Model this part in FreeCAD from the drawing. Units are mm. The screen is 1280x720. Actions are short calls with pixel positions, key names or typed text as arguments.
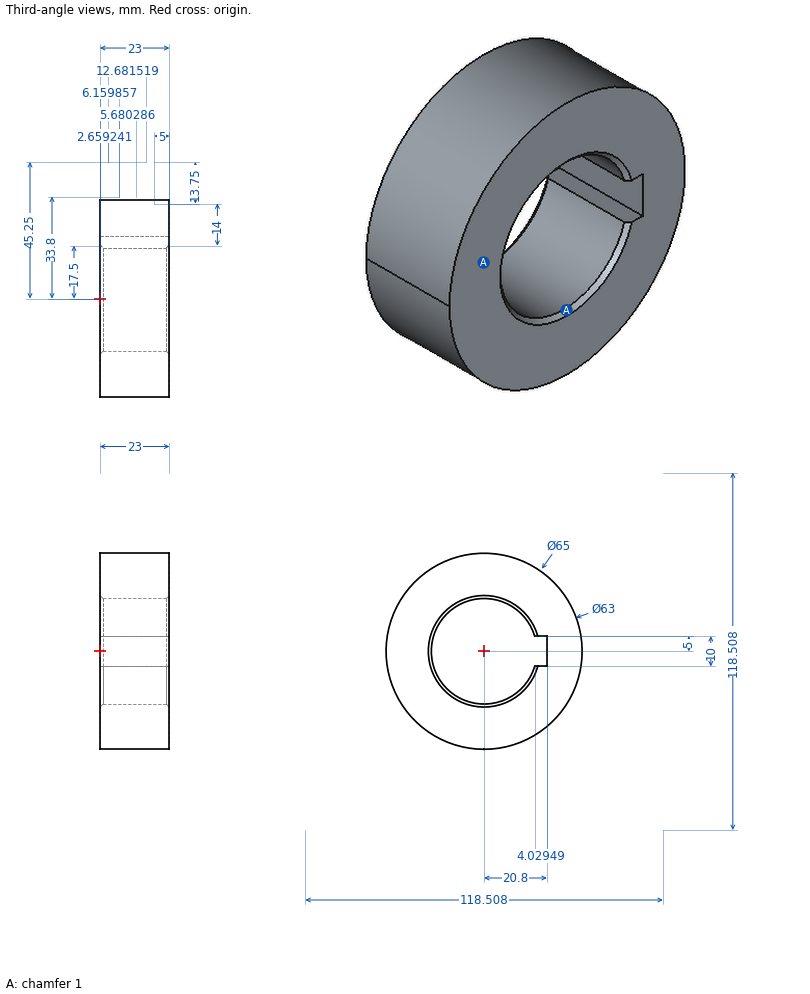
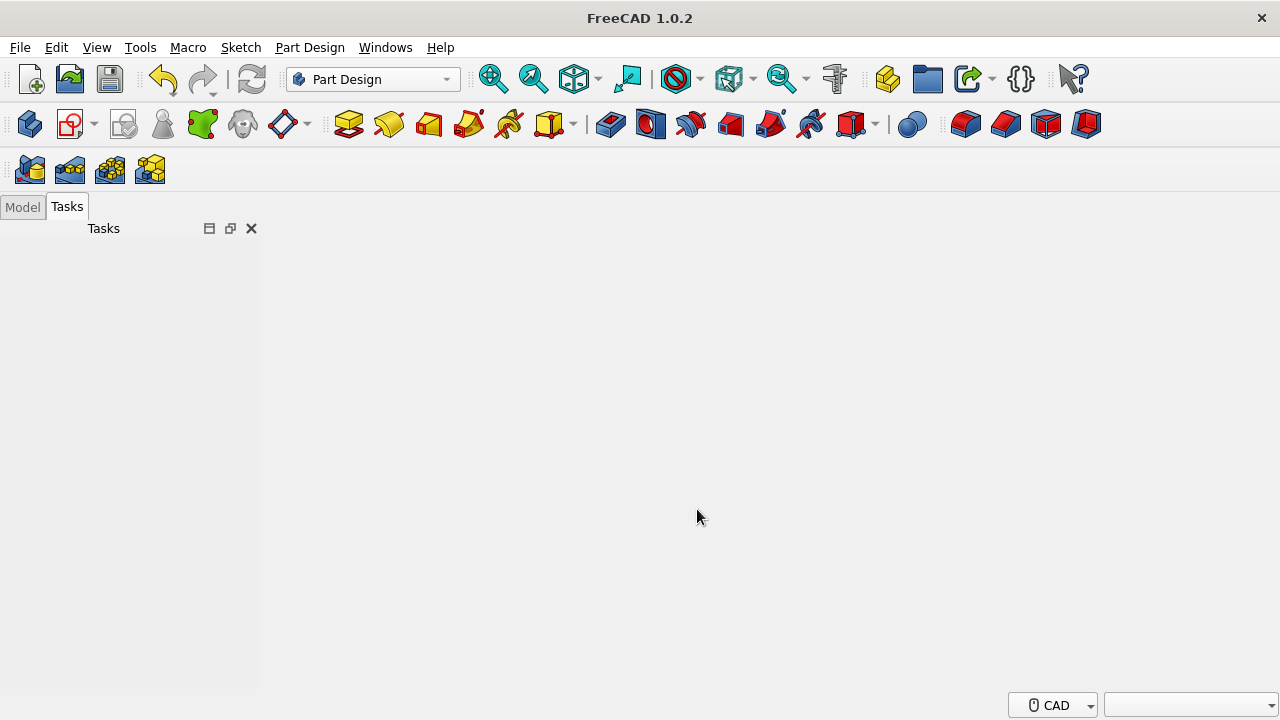
click(30, 80)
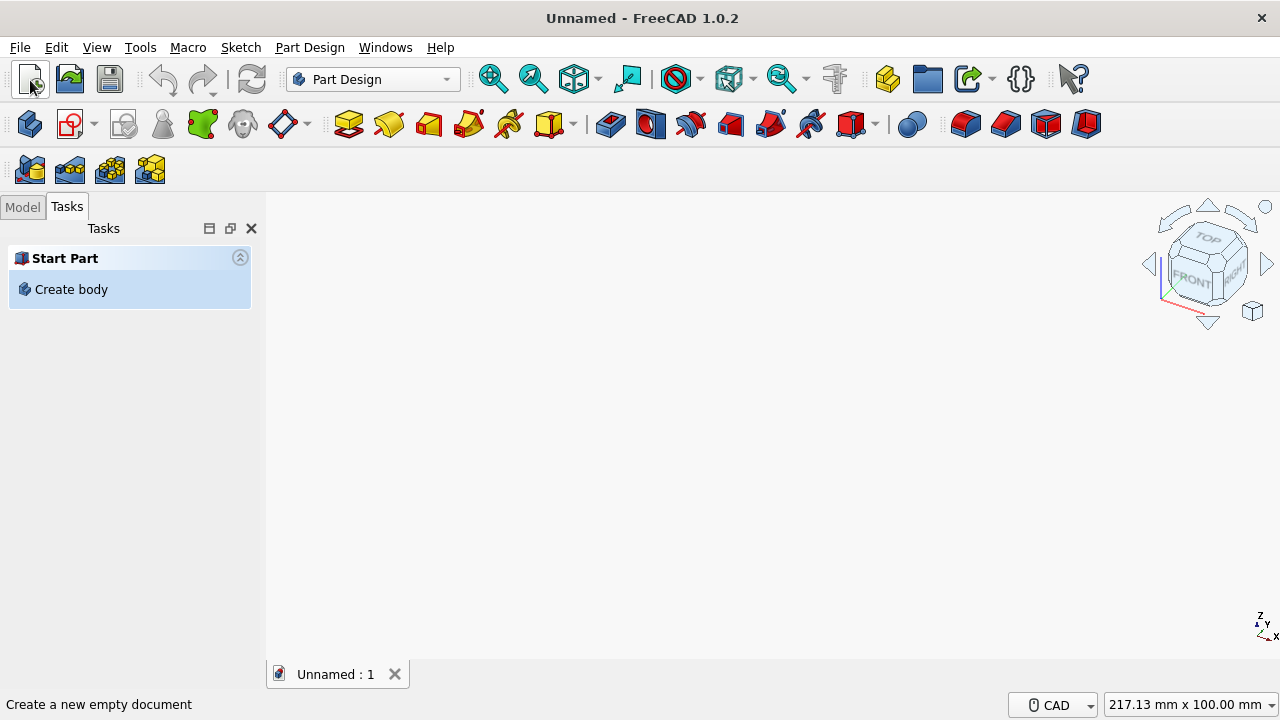
click(70, 124)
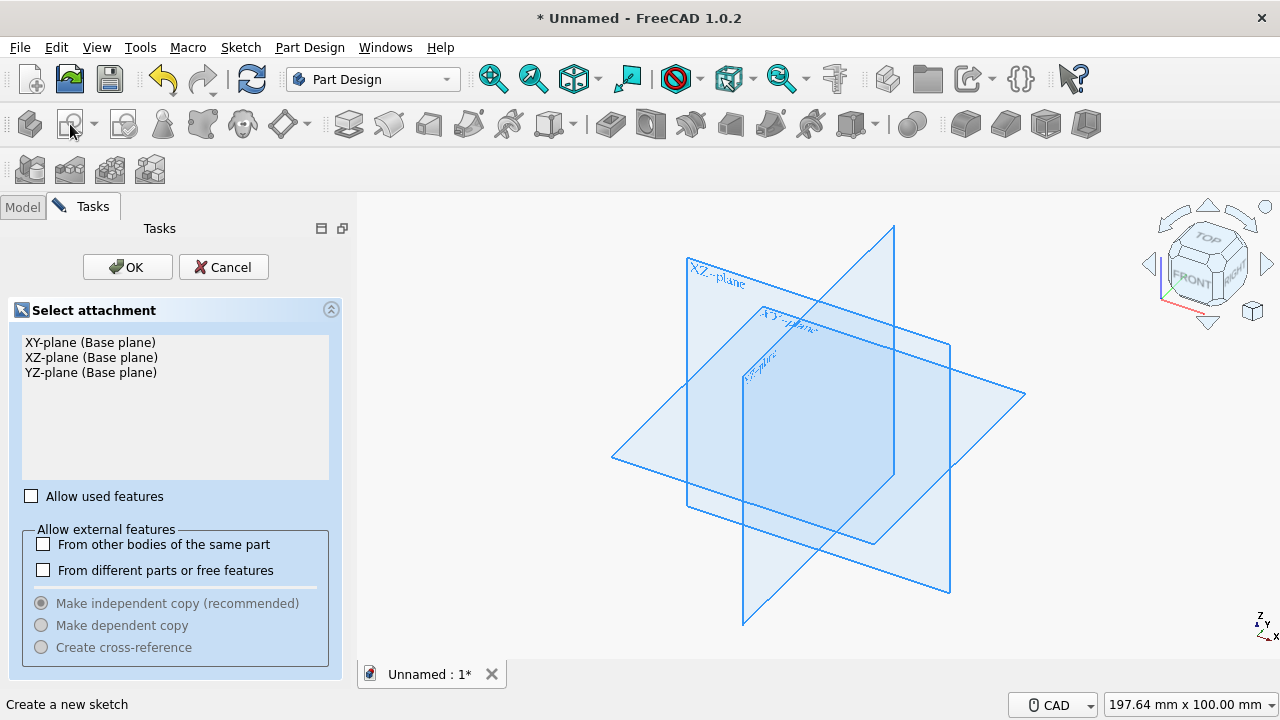
click(82, 342)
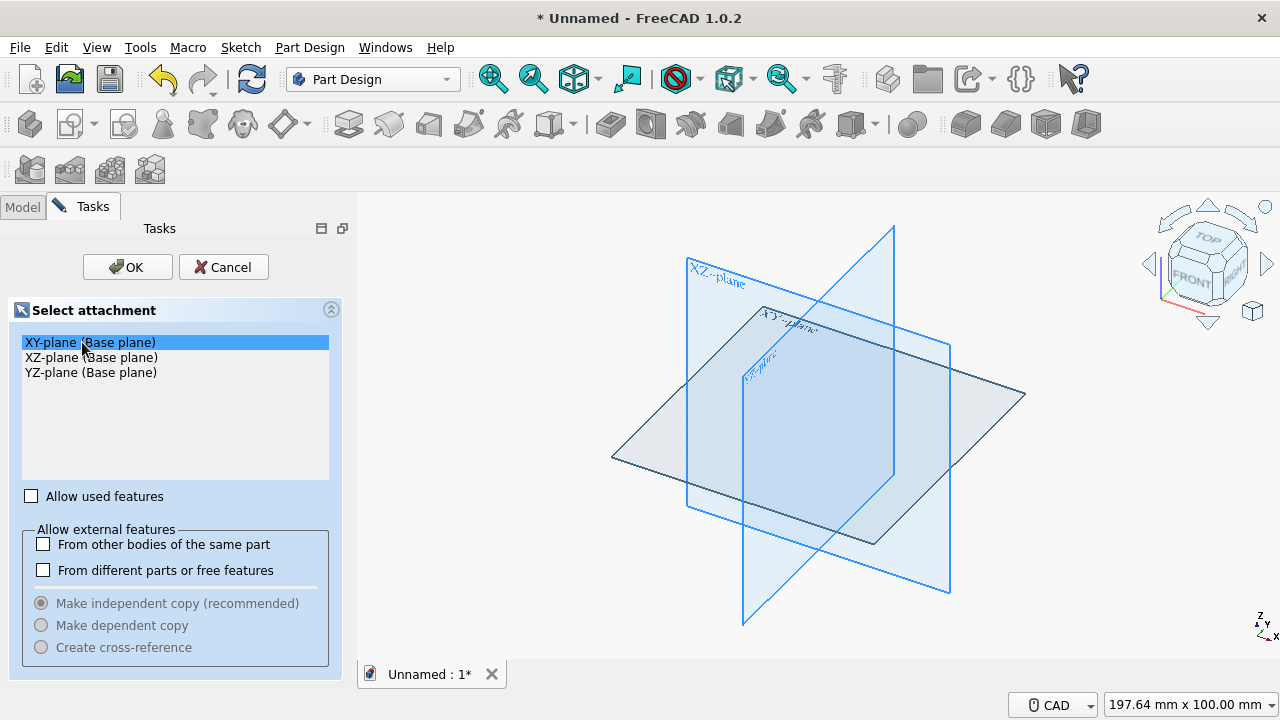
click(128, 267)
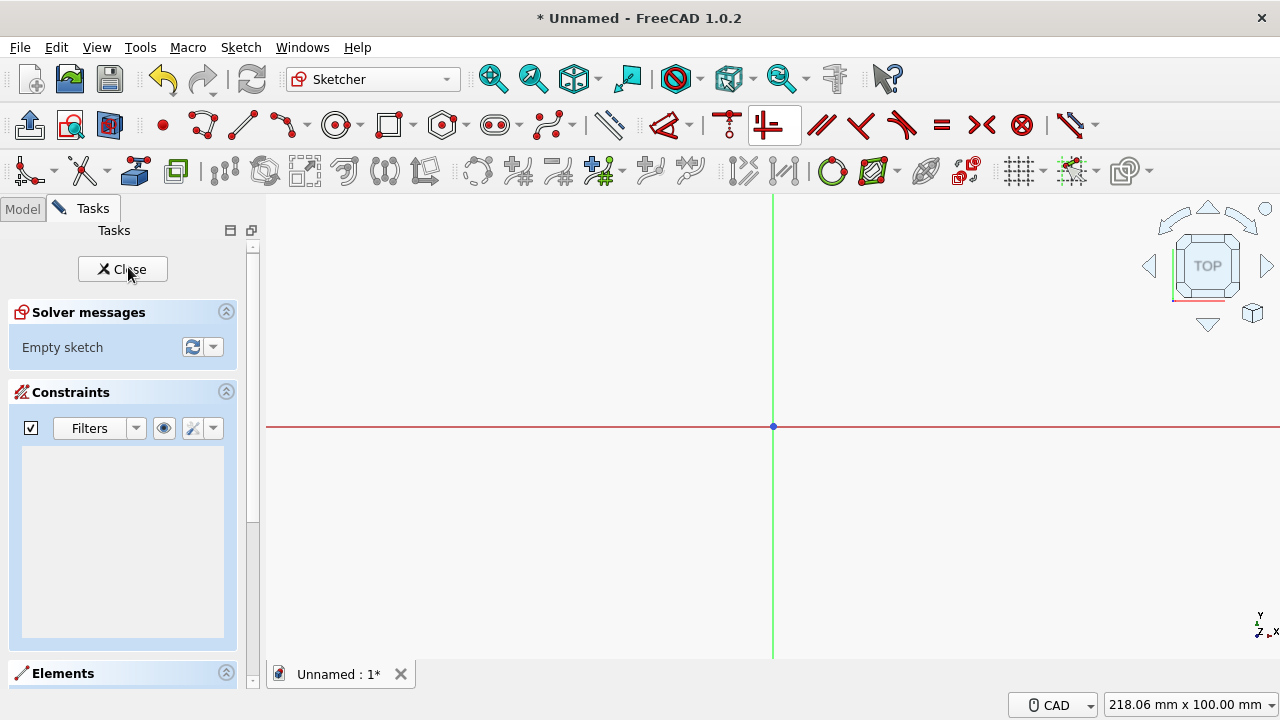
scroll(294, 631, down, 1)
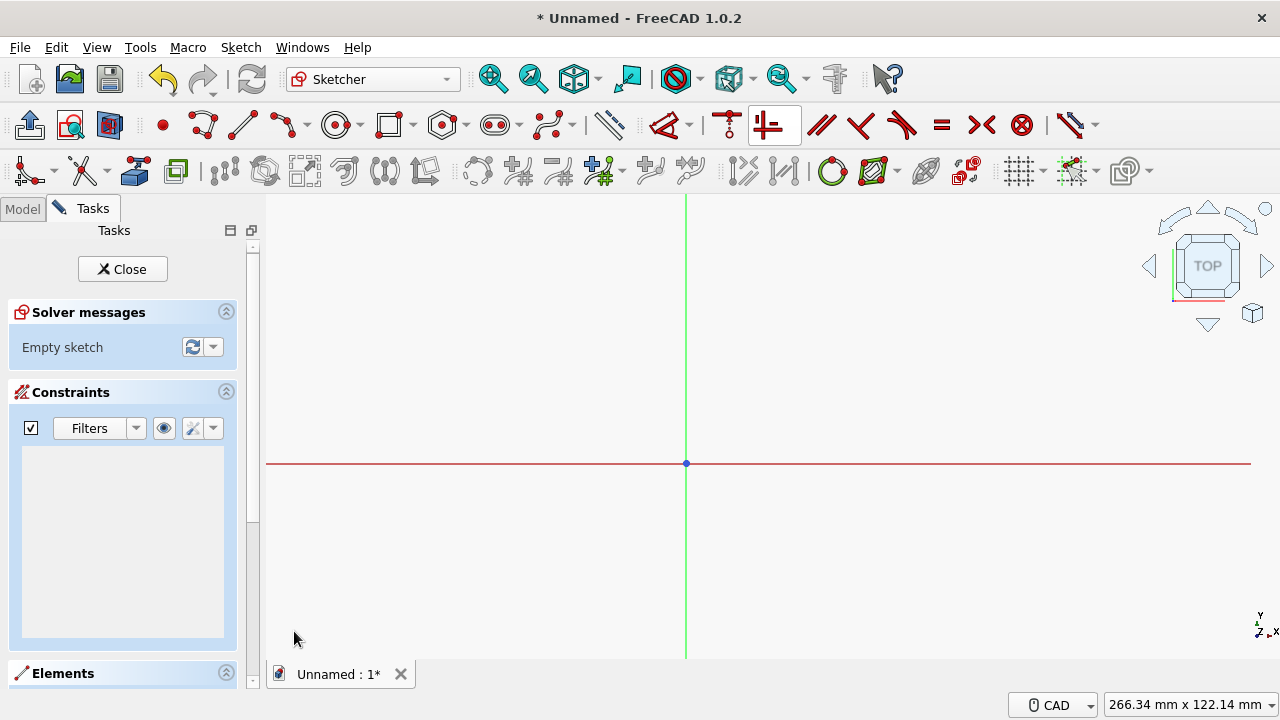
scroll(761, 318, up, 3)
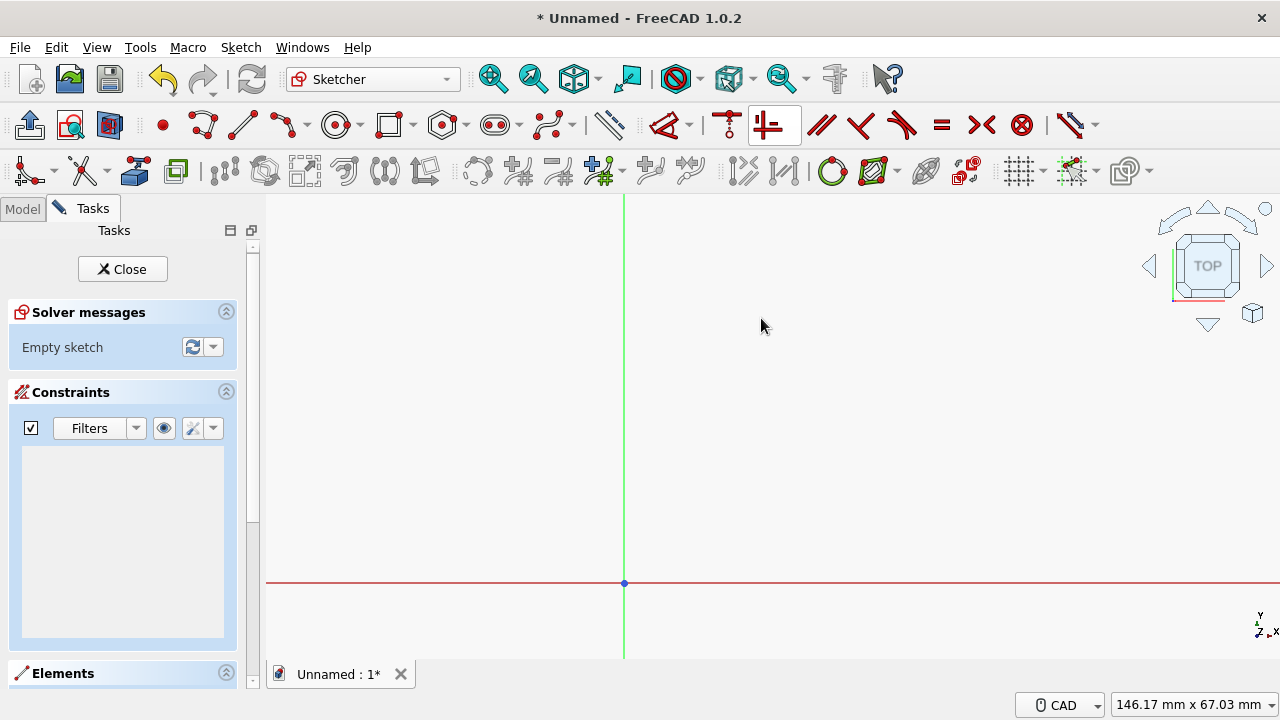
key(g)
key(m)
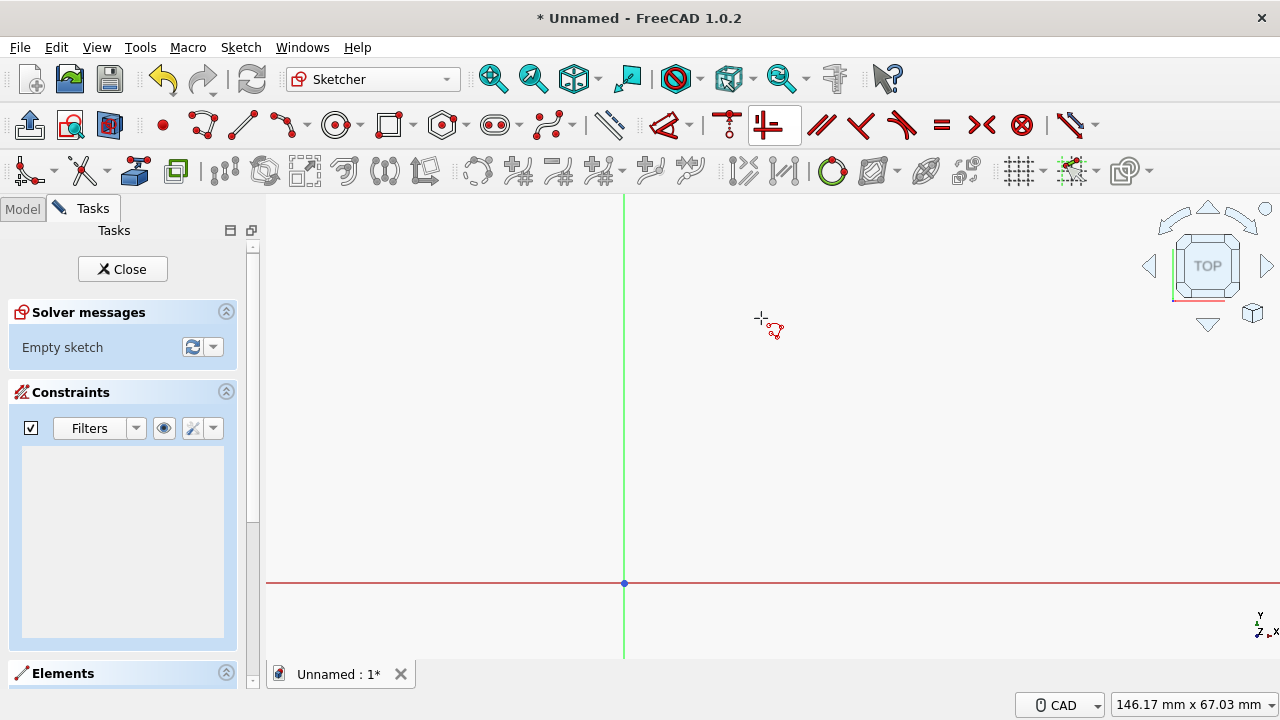
click(624, 462)
click(784, 462)
click(784, 365)
click(749, 365)
click(749, 269)
click(633, 269)
click(624, 463)
key(Escape)
key(Escape)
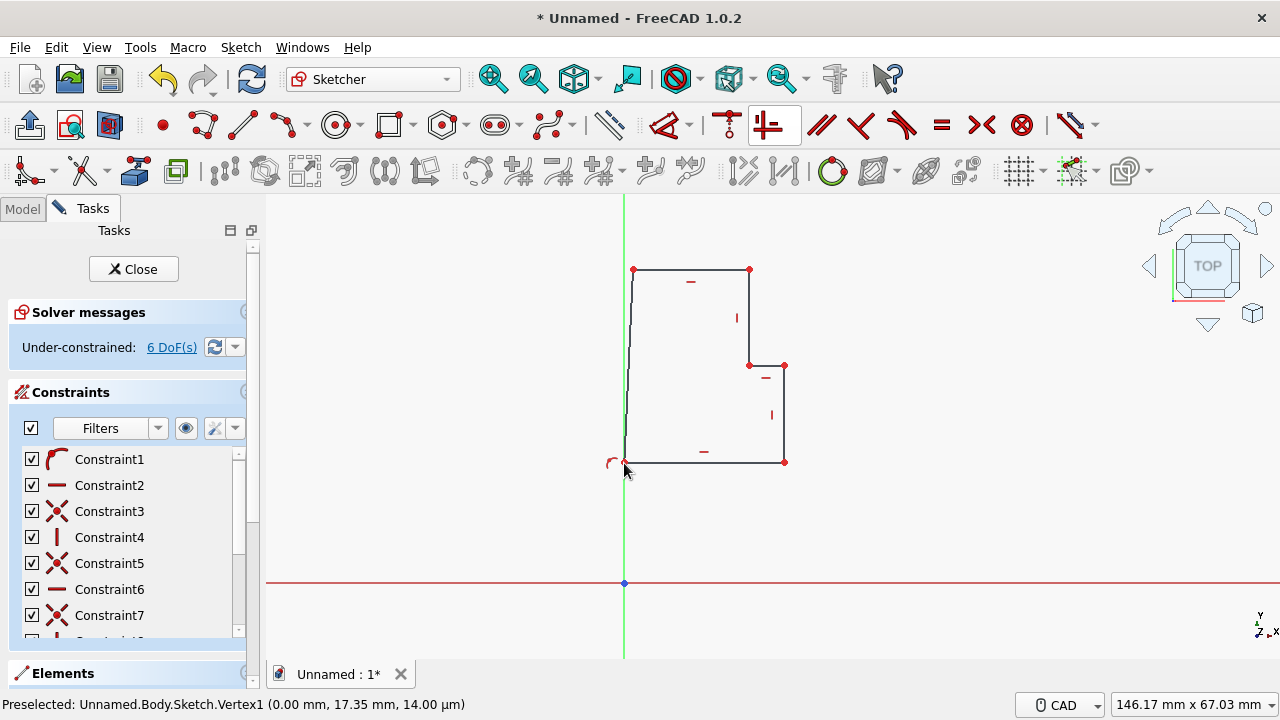
click(627, 405)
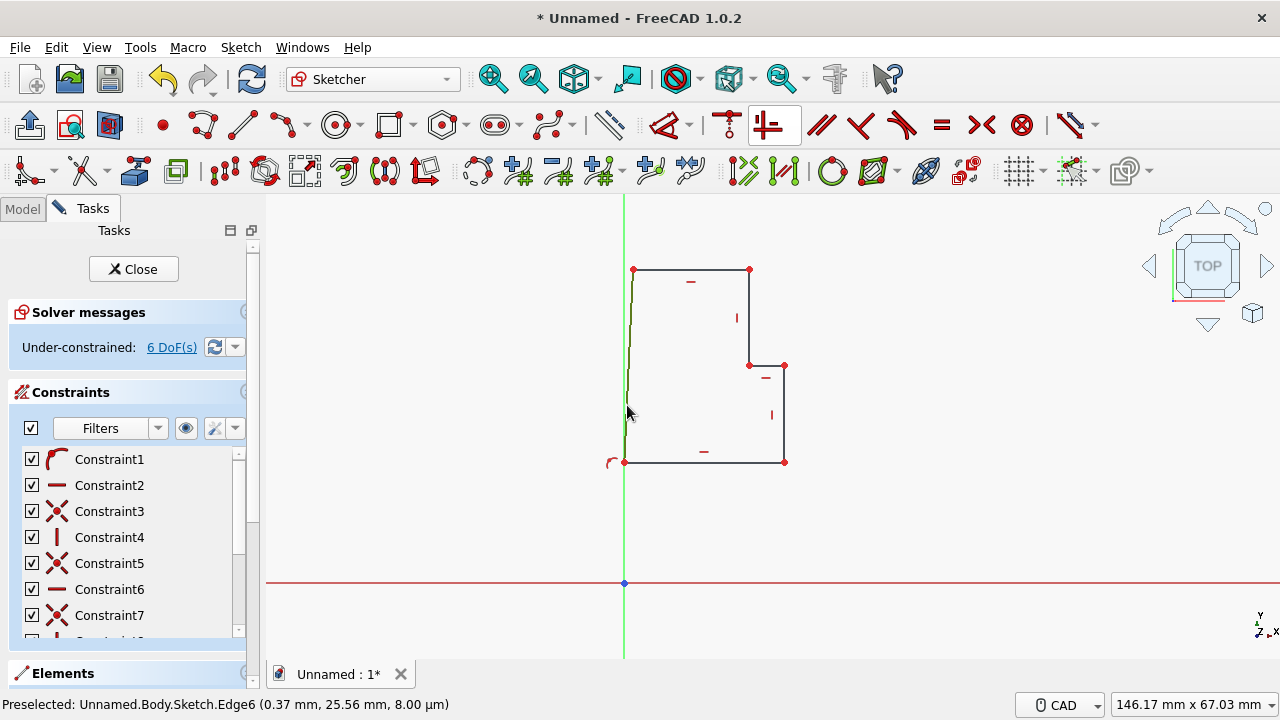
key(v)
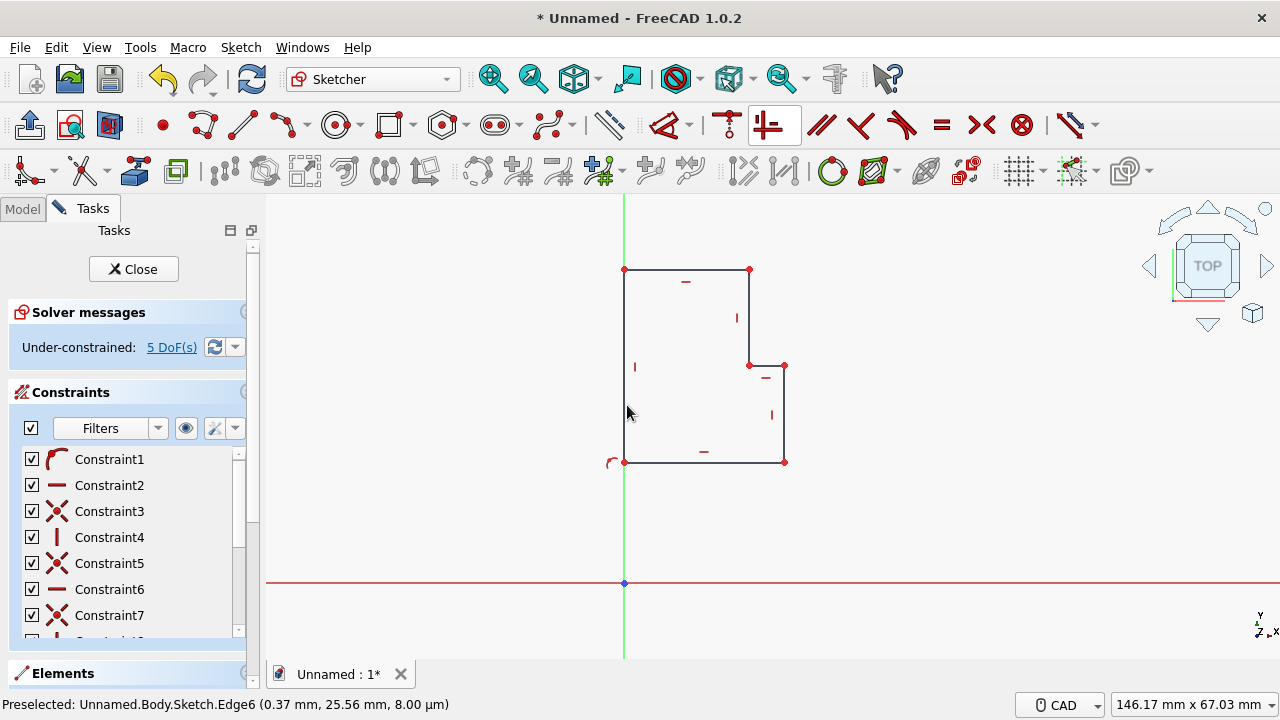
key(d)